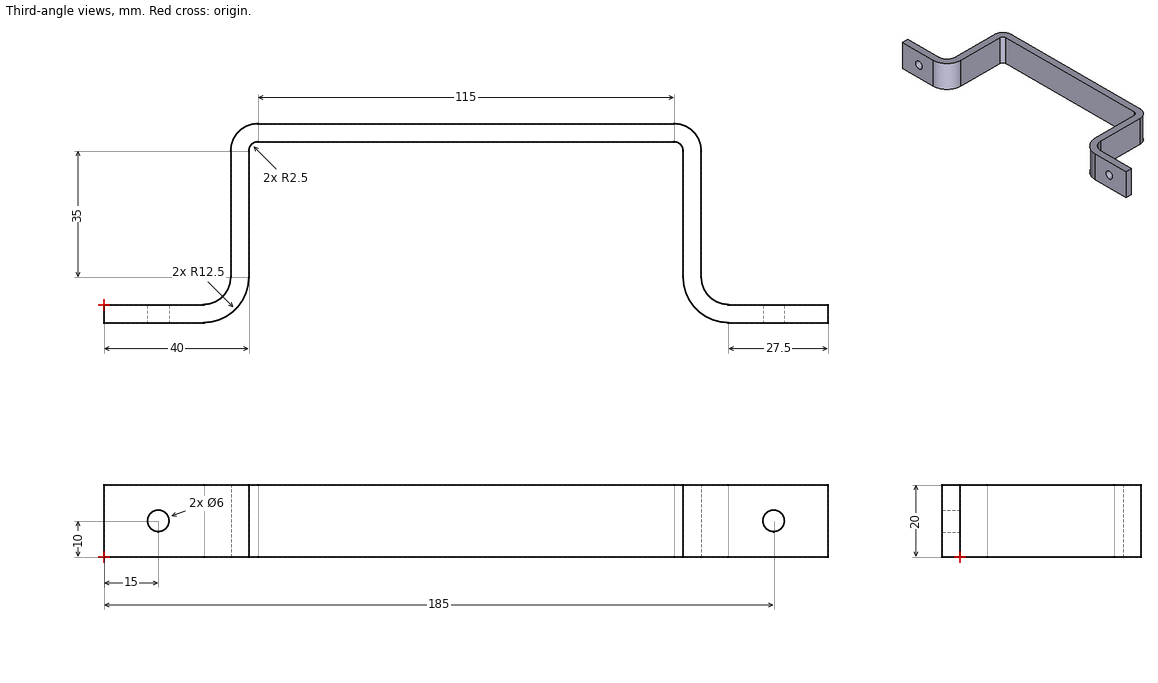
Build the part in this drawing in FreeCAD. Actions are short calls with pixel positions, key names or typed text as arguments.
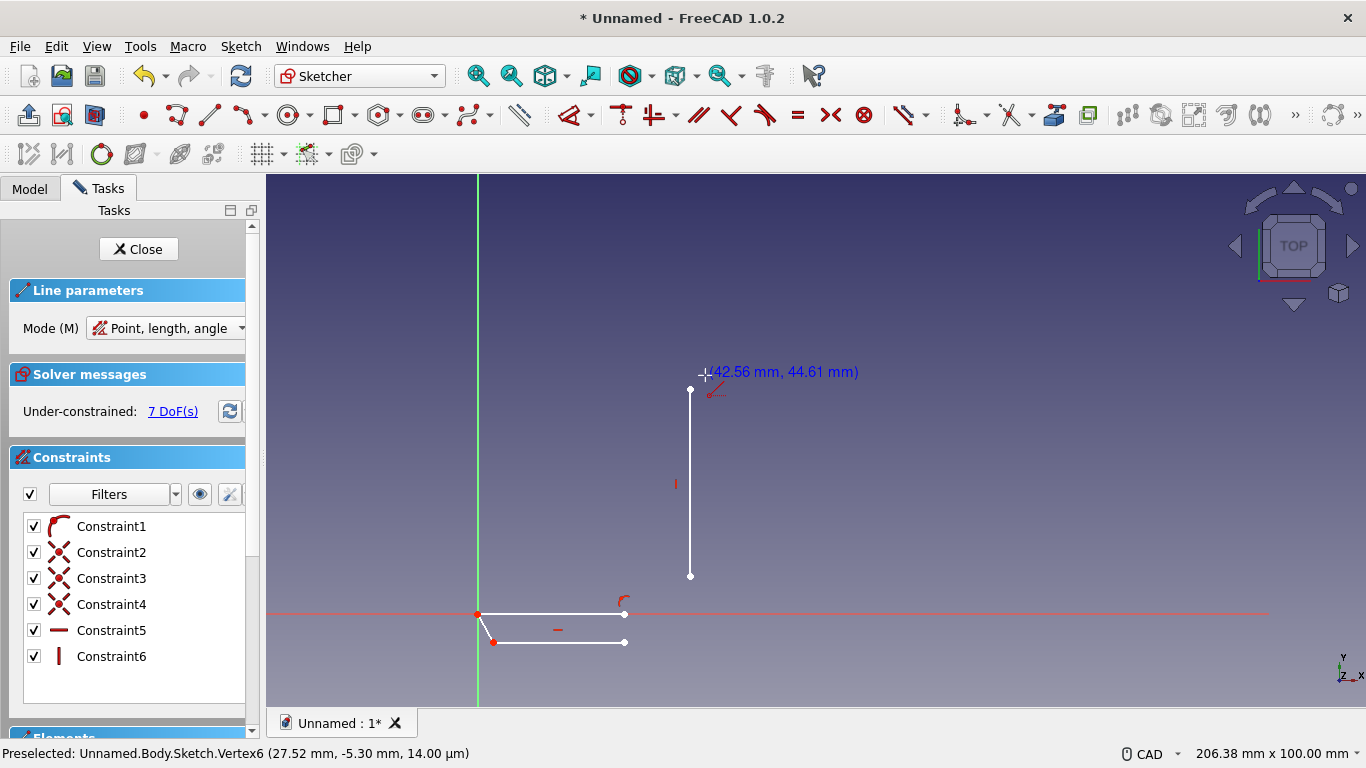
click(704, 374)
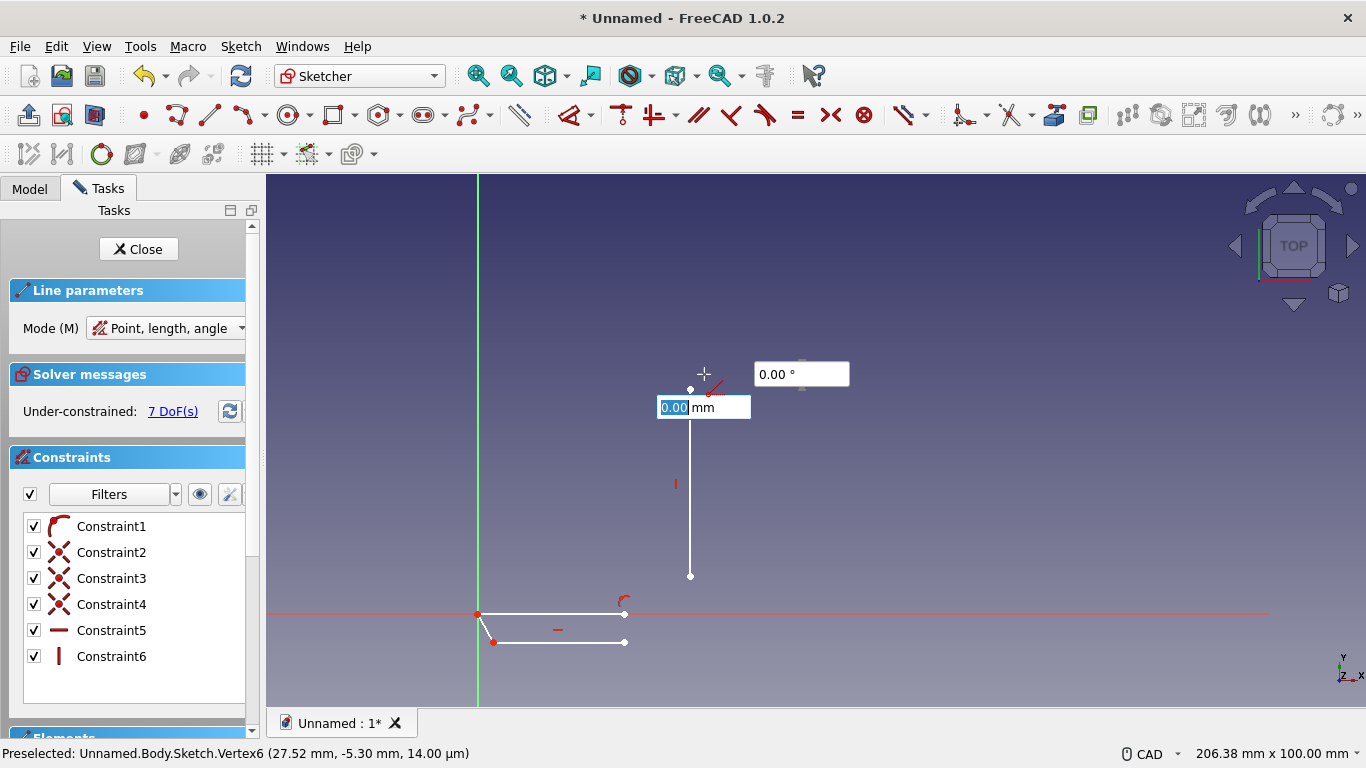
scroll(427, 375, down, 3)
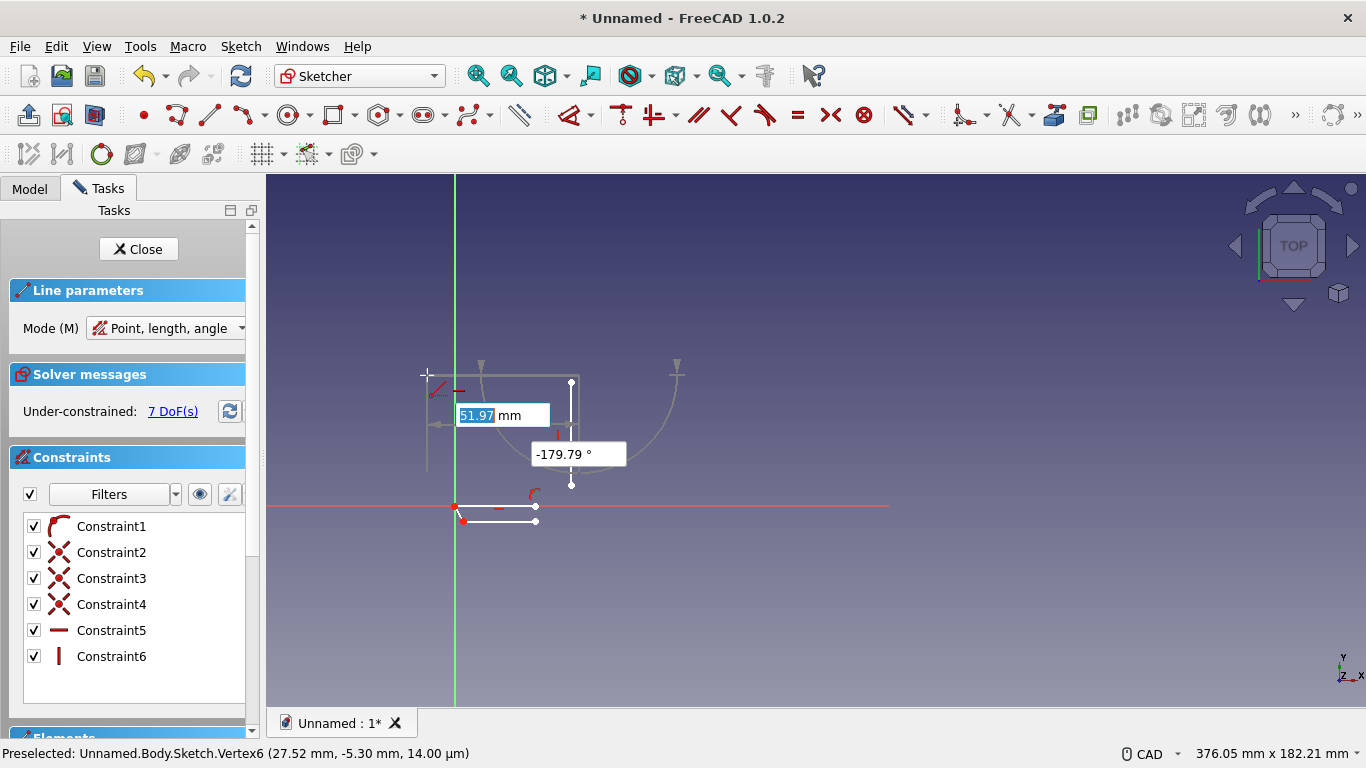
click(916, 375)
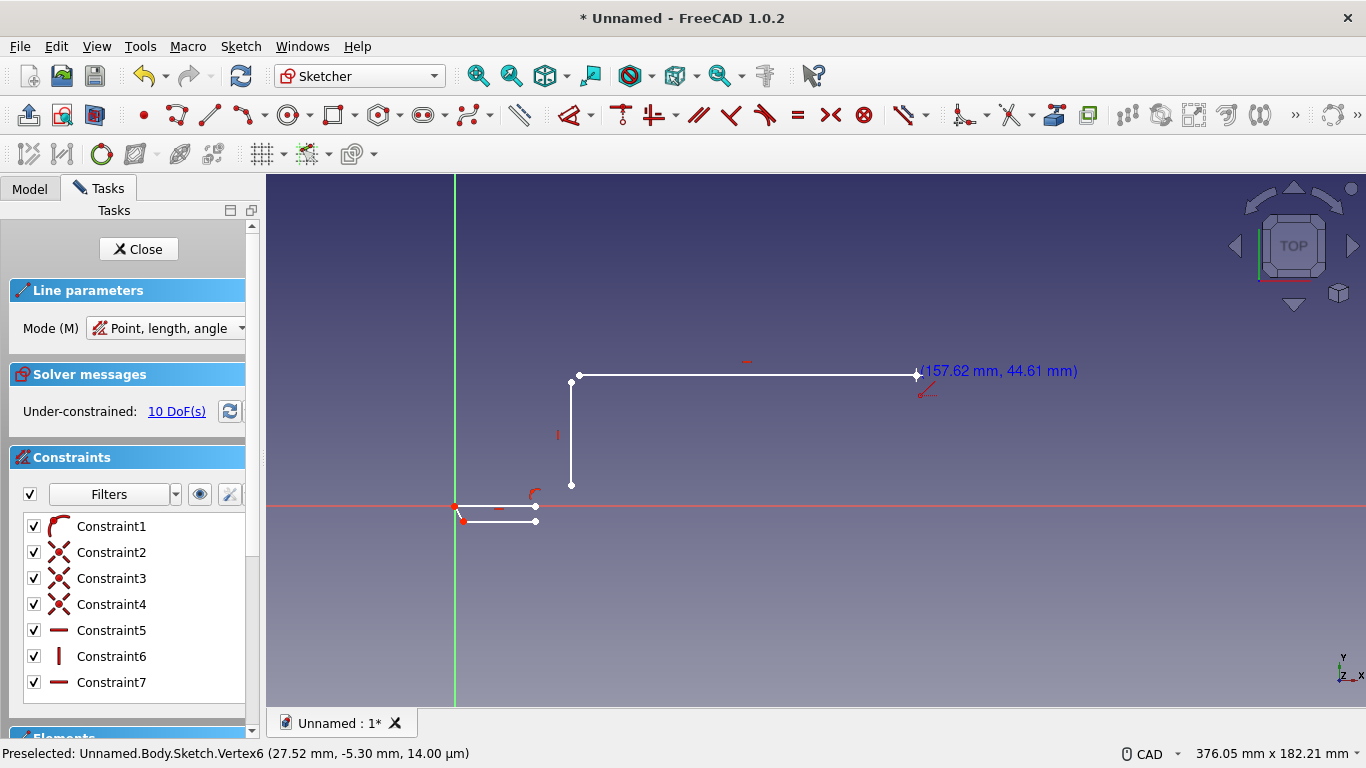
scroll(923, 382, up, 3)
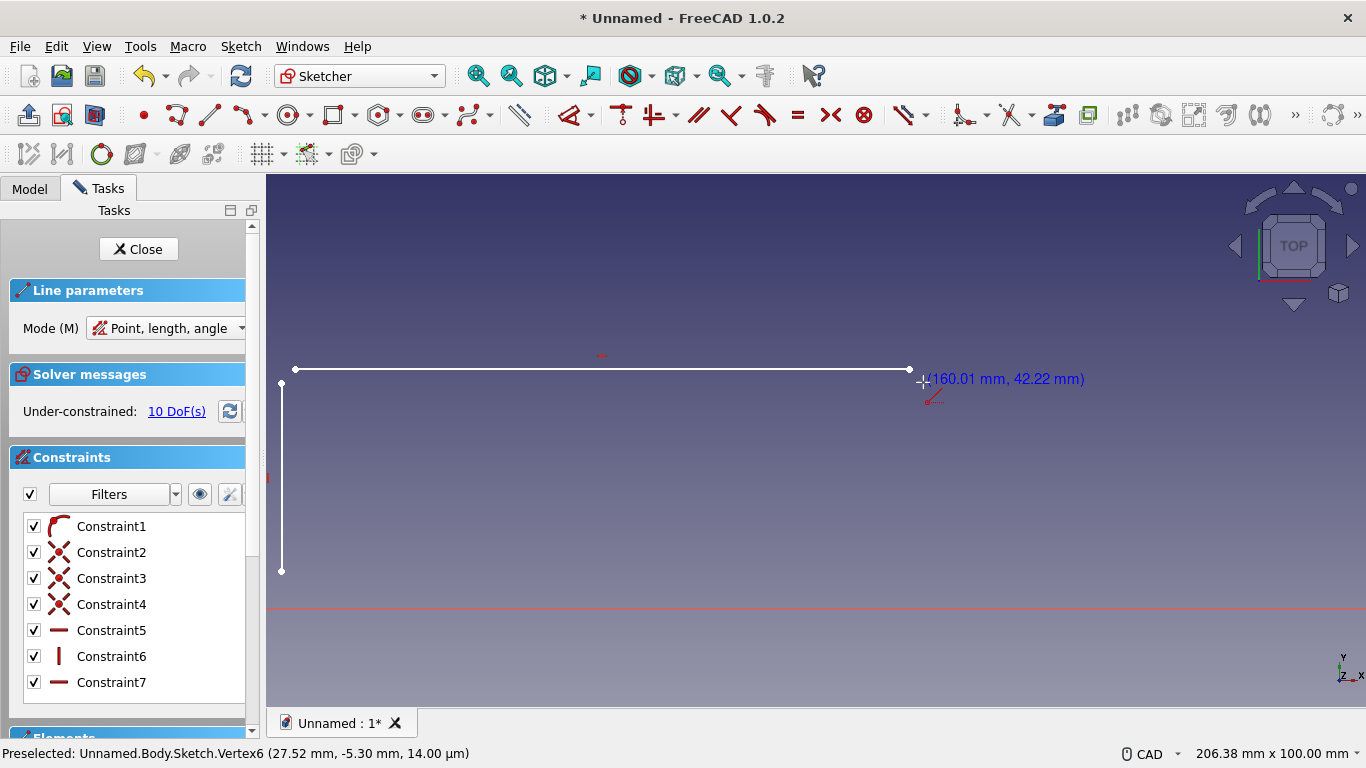
click(922, 382)
click(922, 569)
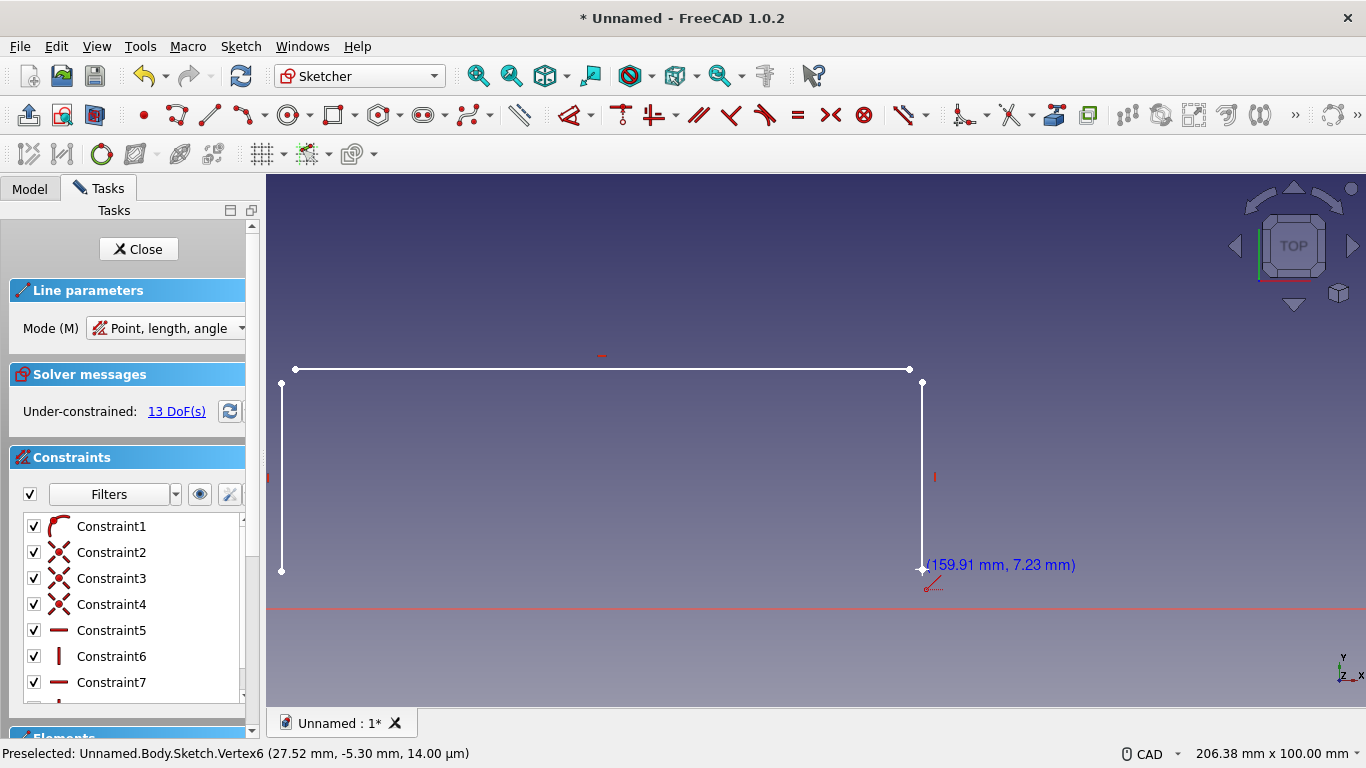
click(177, 116)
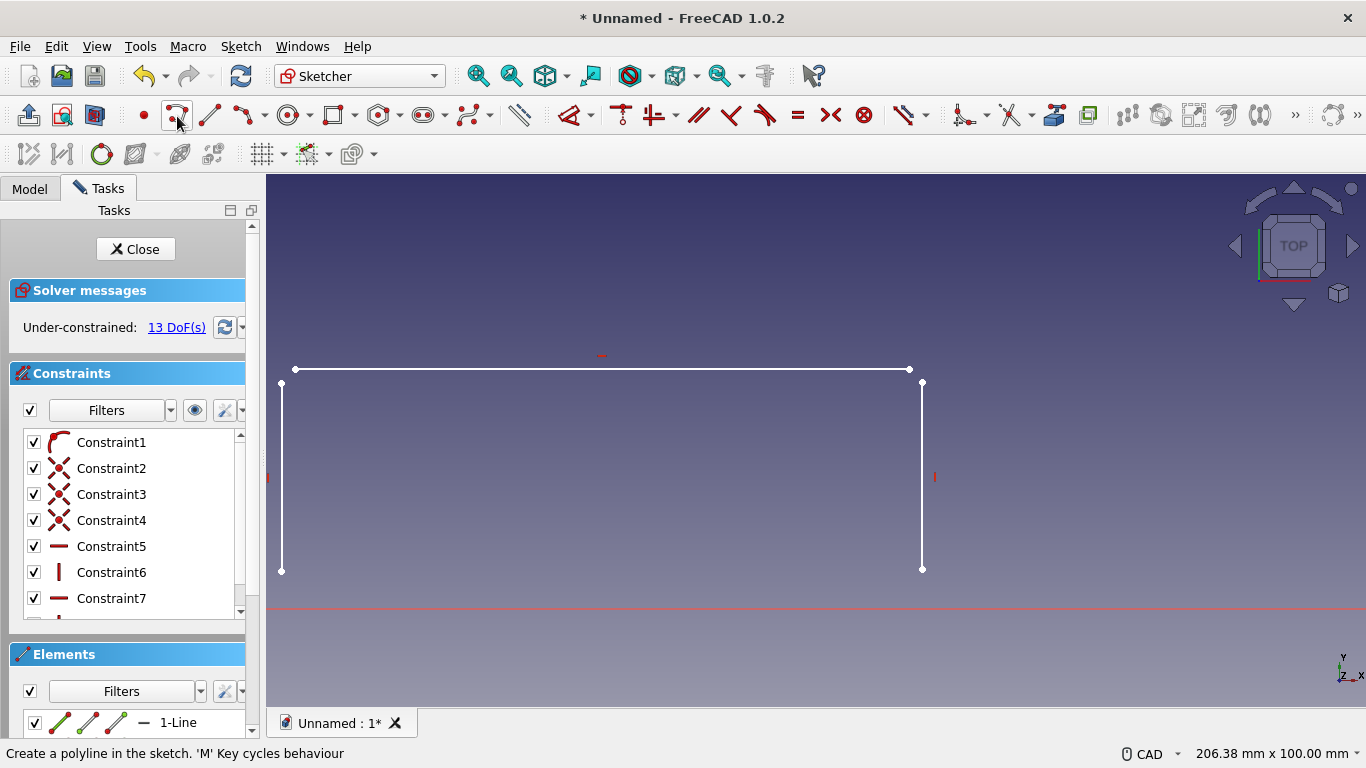
click(989, 635)
click(1136, 635)
click(1136, 609)
click(989, 600)
right_click(989, 600)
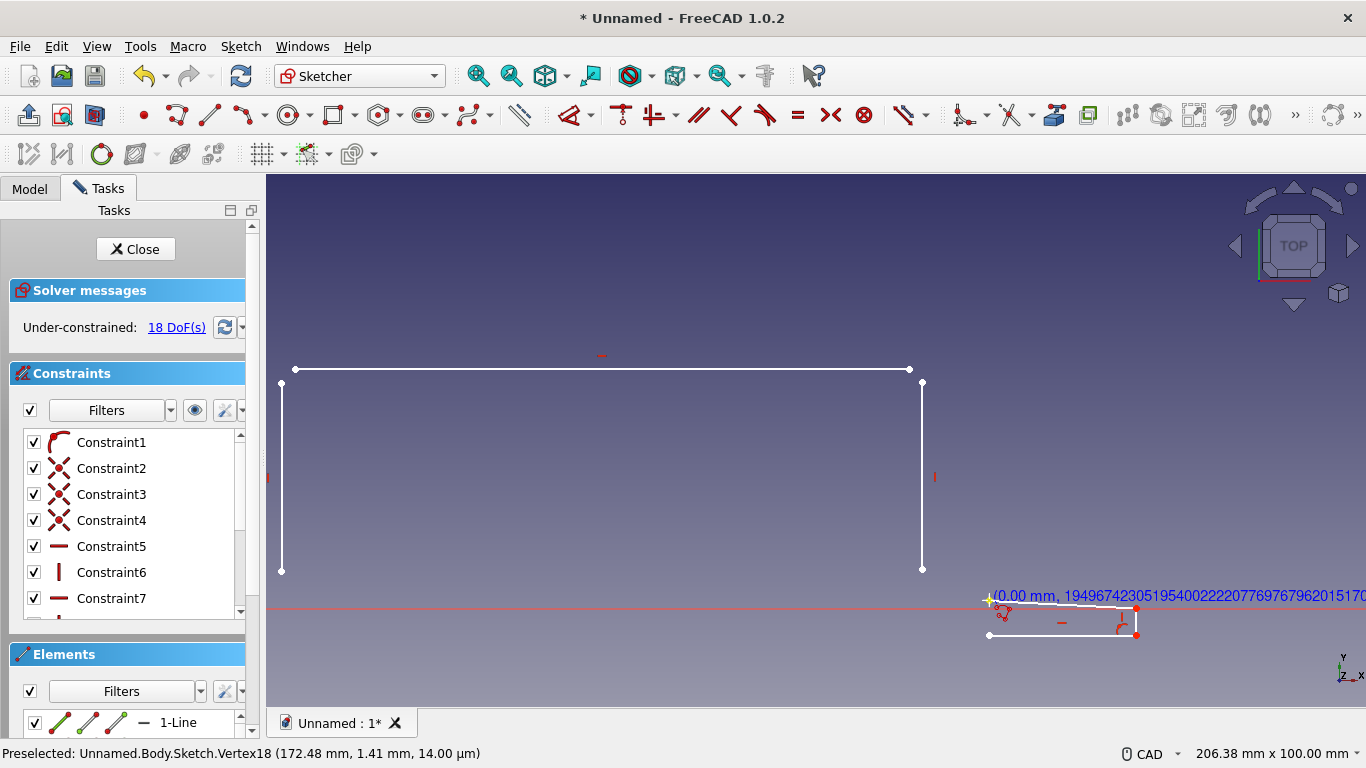
key(g)
key(l)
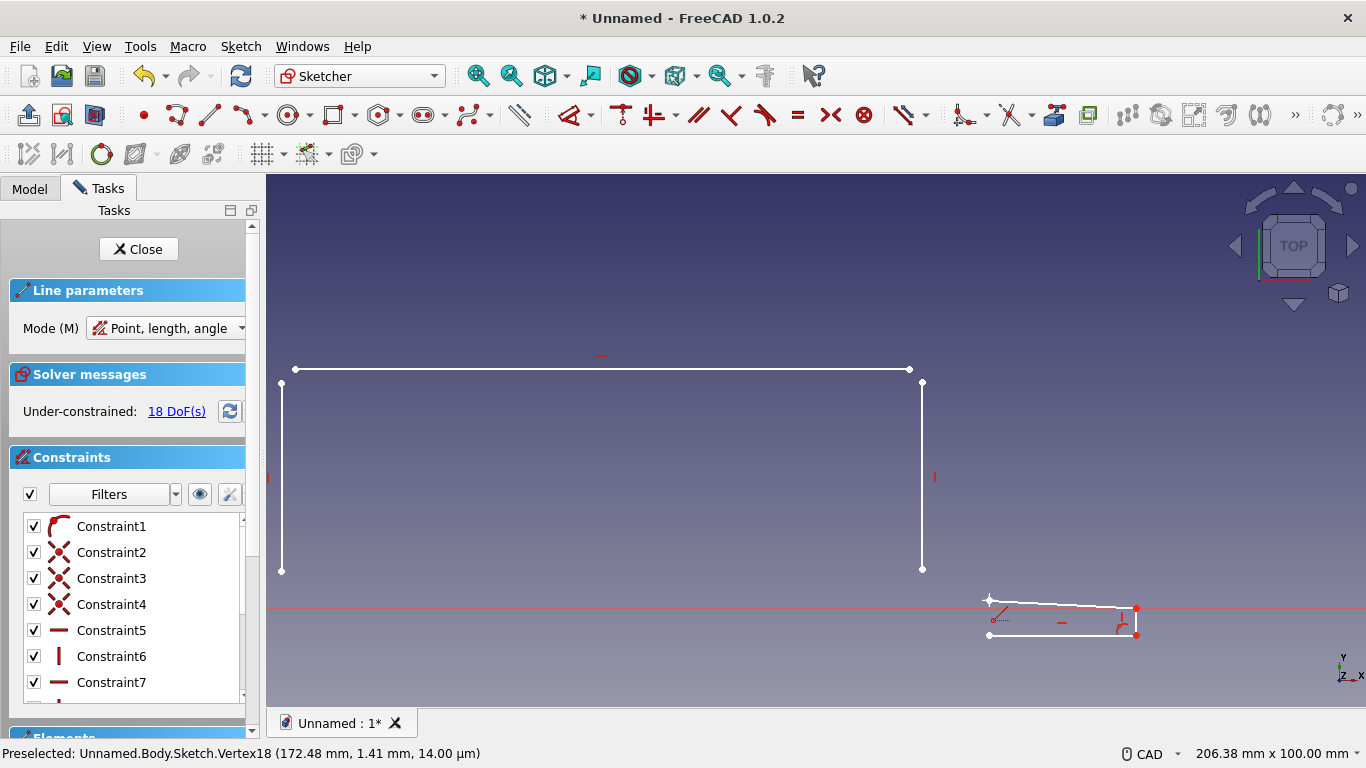
click(949, 569)
click(949, 382)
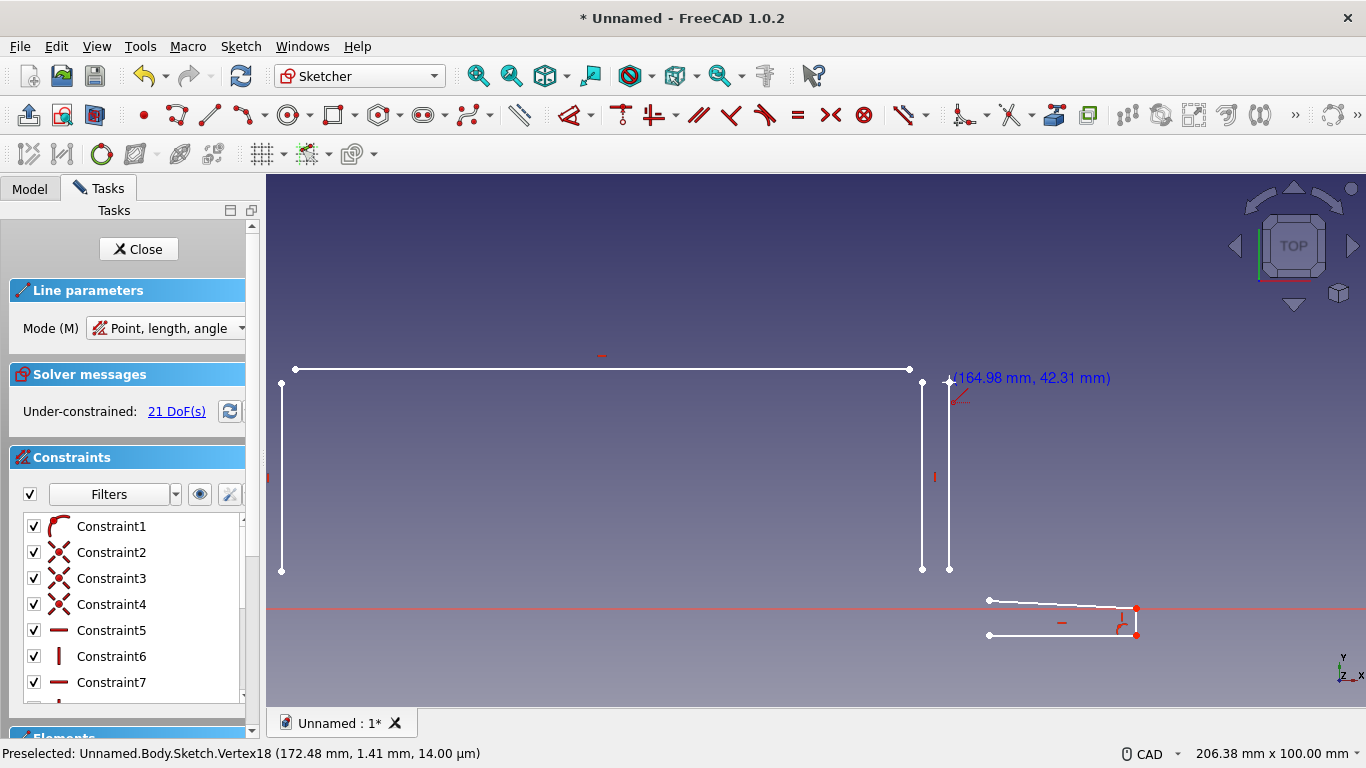
click(909, 342)
click(296, 342)